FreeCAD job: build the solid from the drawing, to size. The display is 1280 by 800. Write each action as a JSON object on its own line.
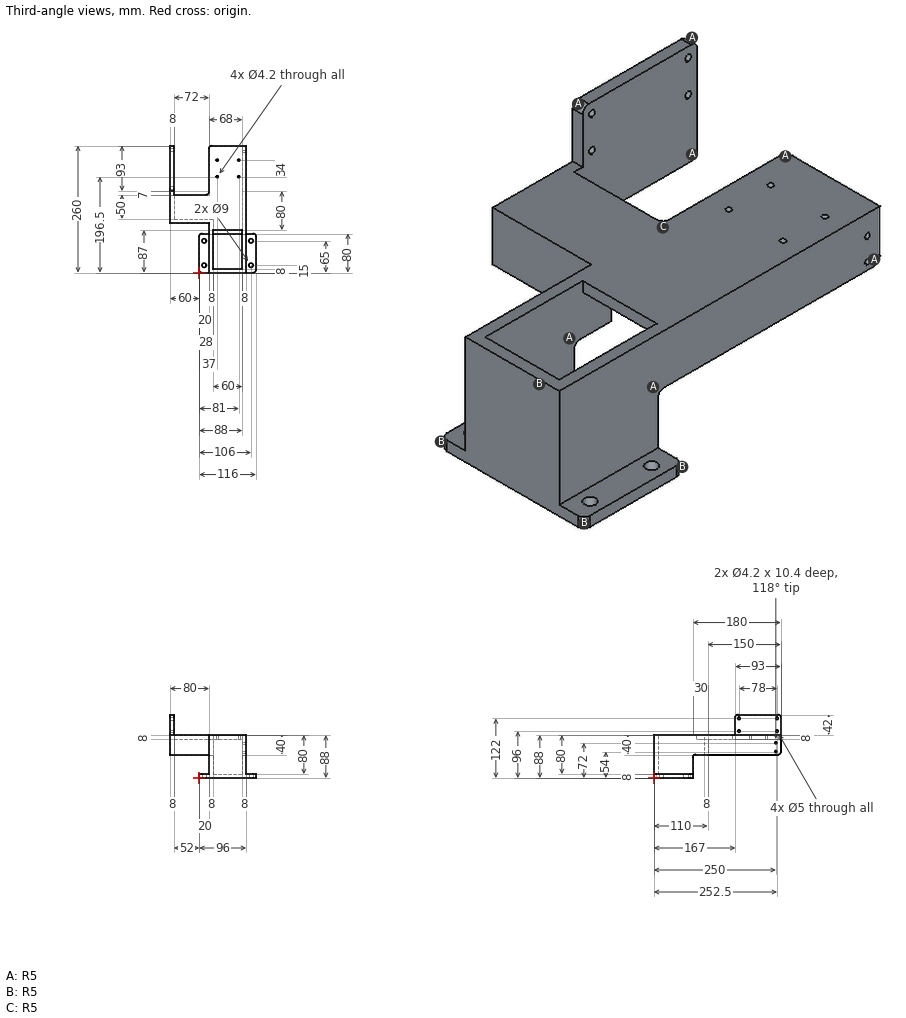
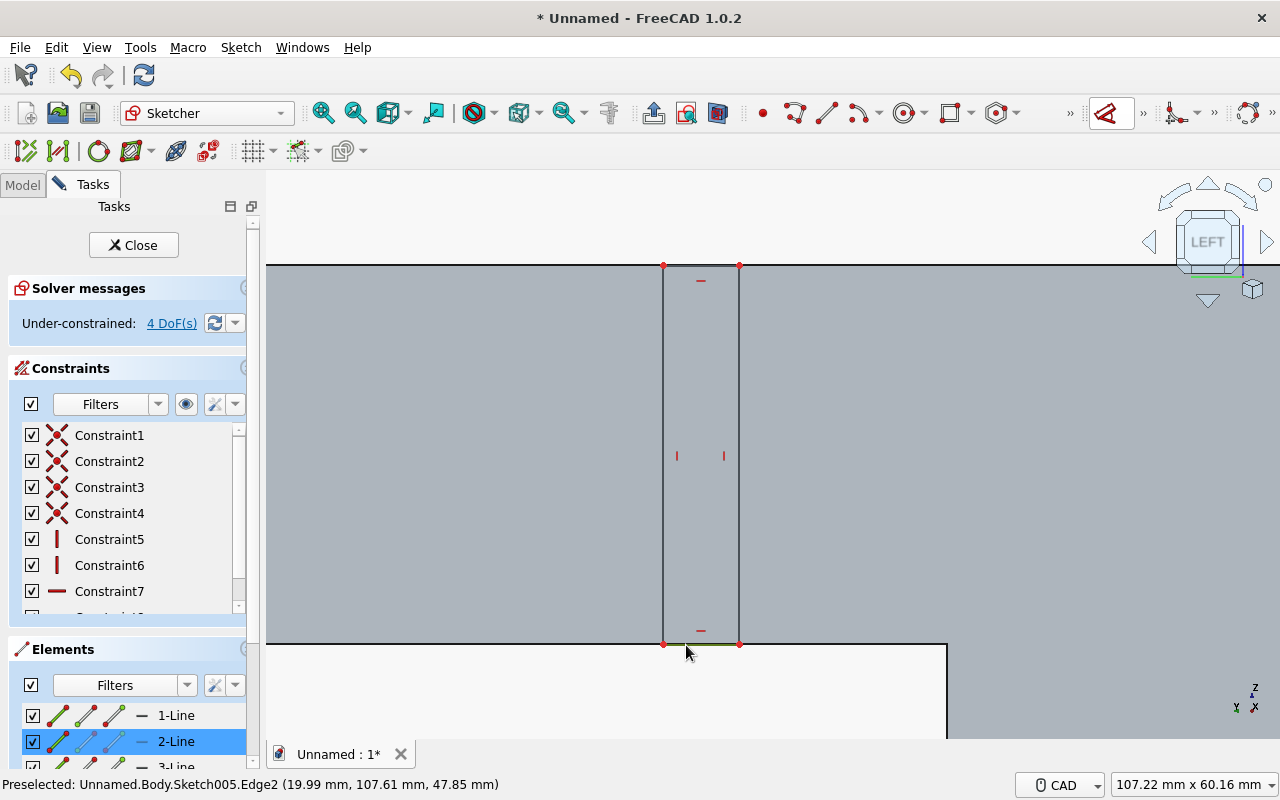
{"action": "left_click", "coordinate": [1128, 114]}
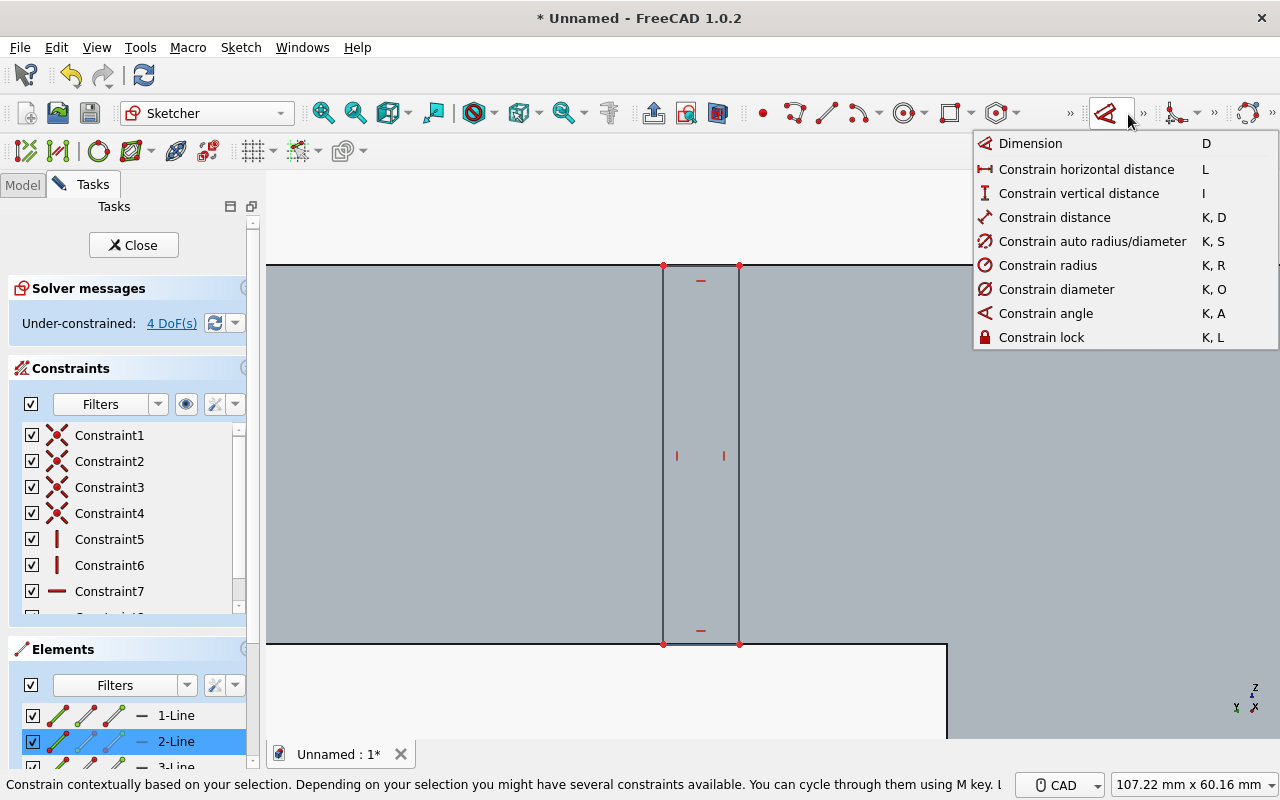
{"action": "left_click", "coordinate": [1126, 169]}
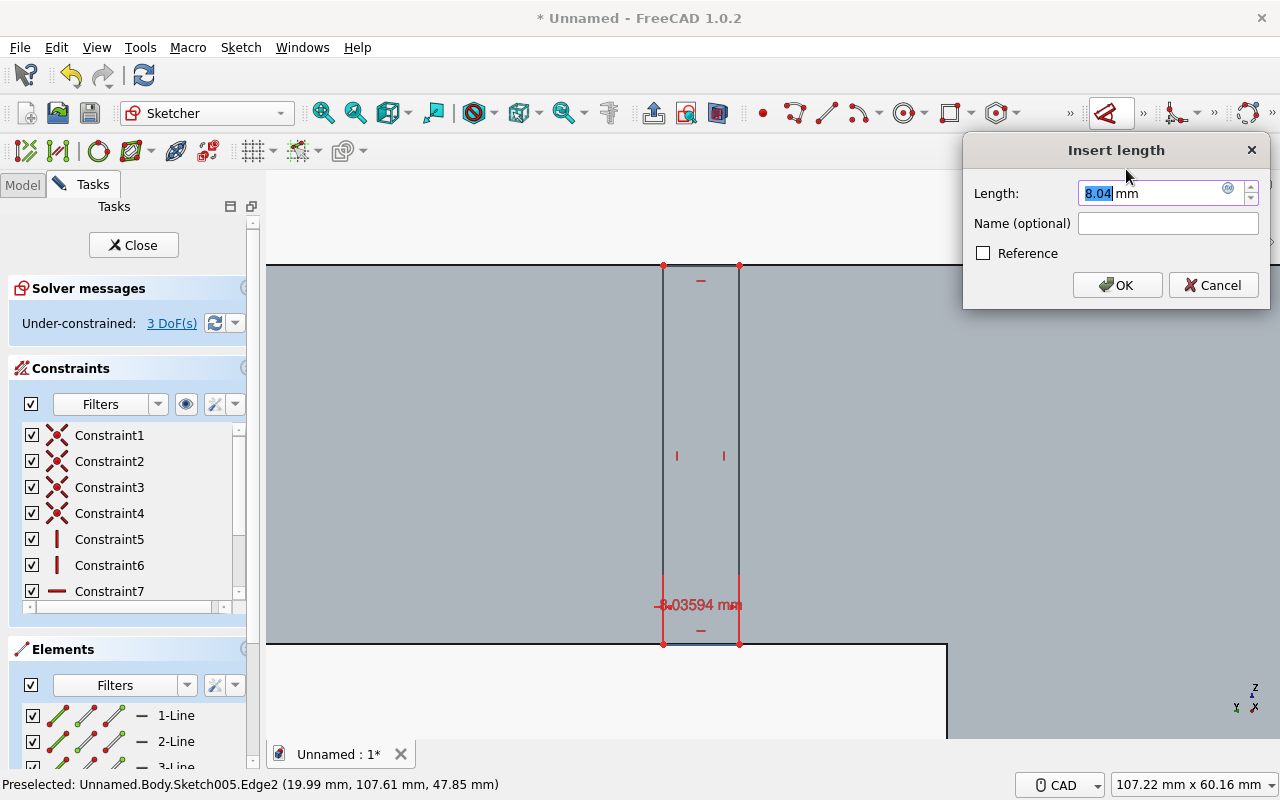
{"action": "type", "text": "8"}
{"action": "key", "text": "Return"}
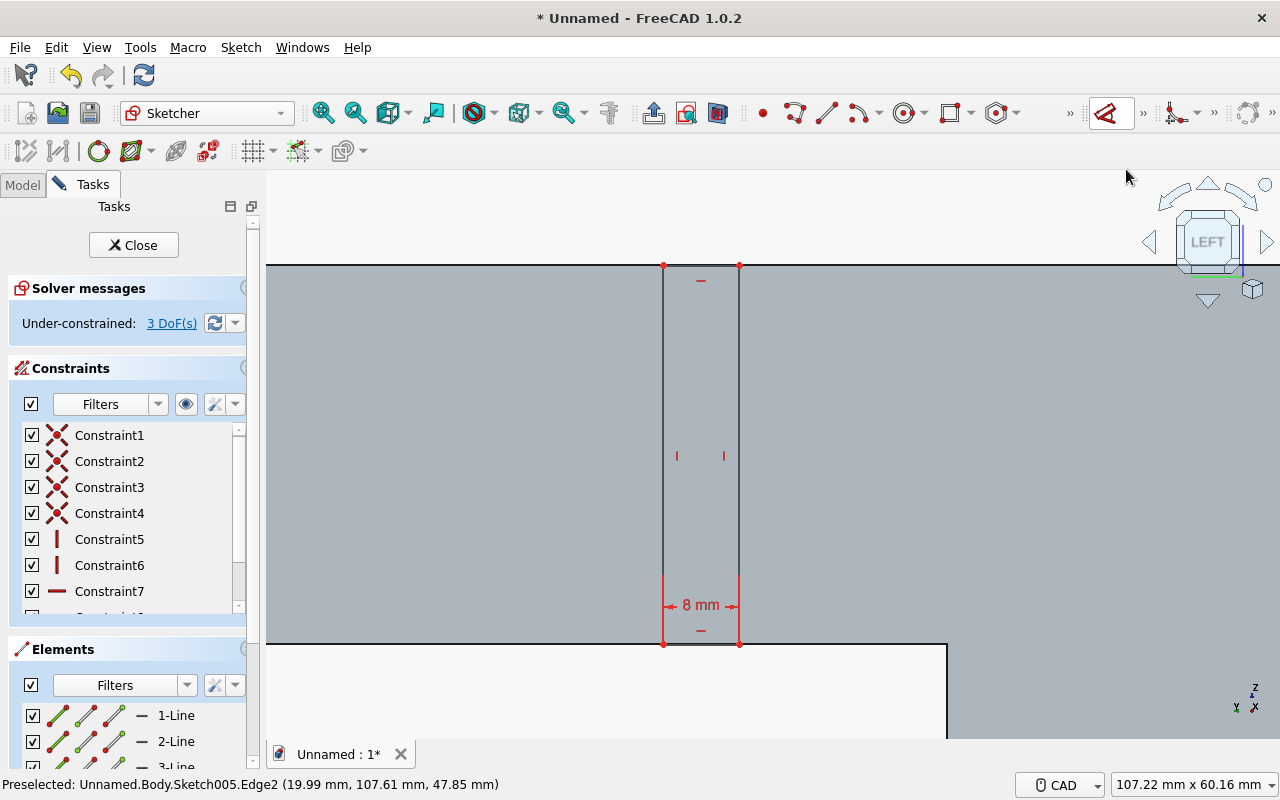
{"action": "left_click", "coordinate": [663, 380]}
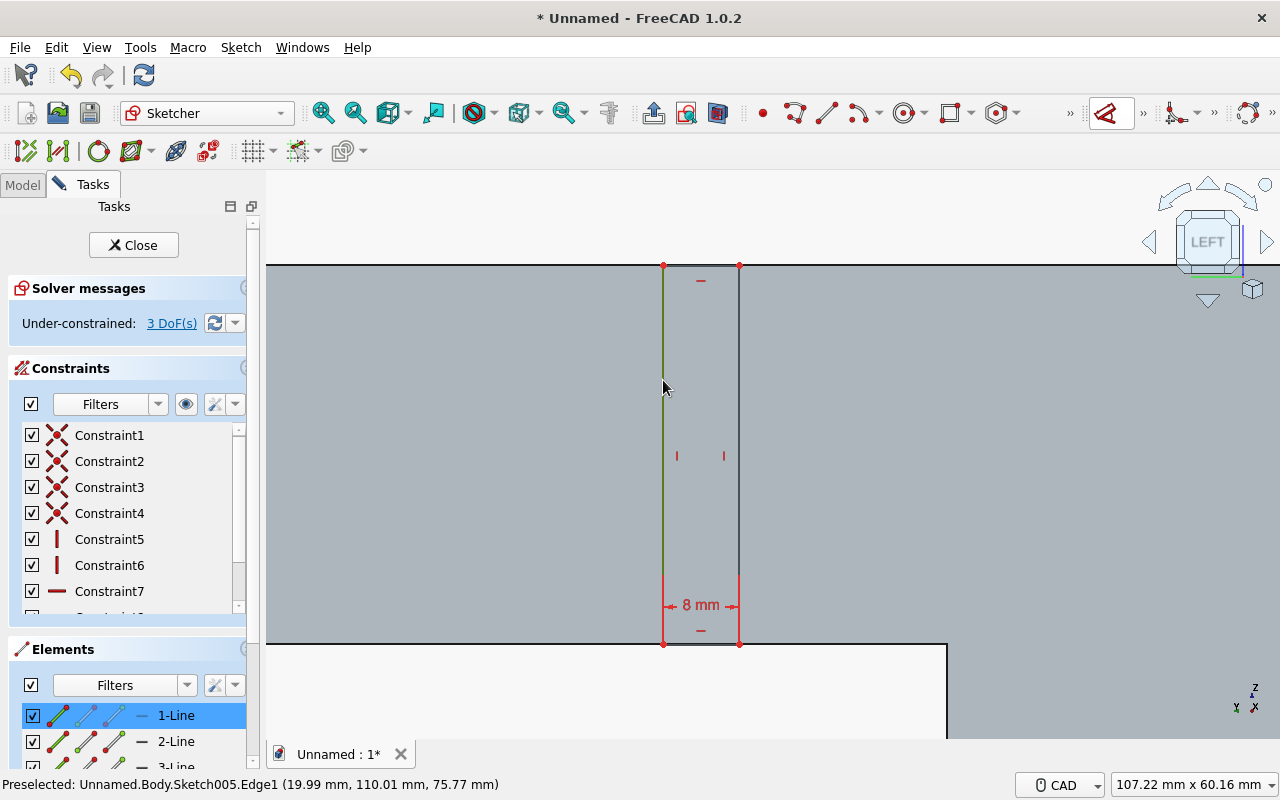
{"action": "left_click", "coordinate": [1128, 114]}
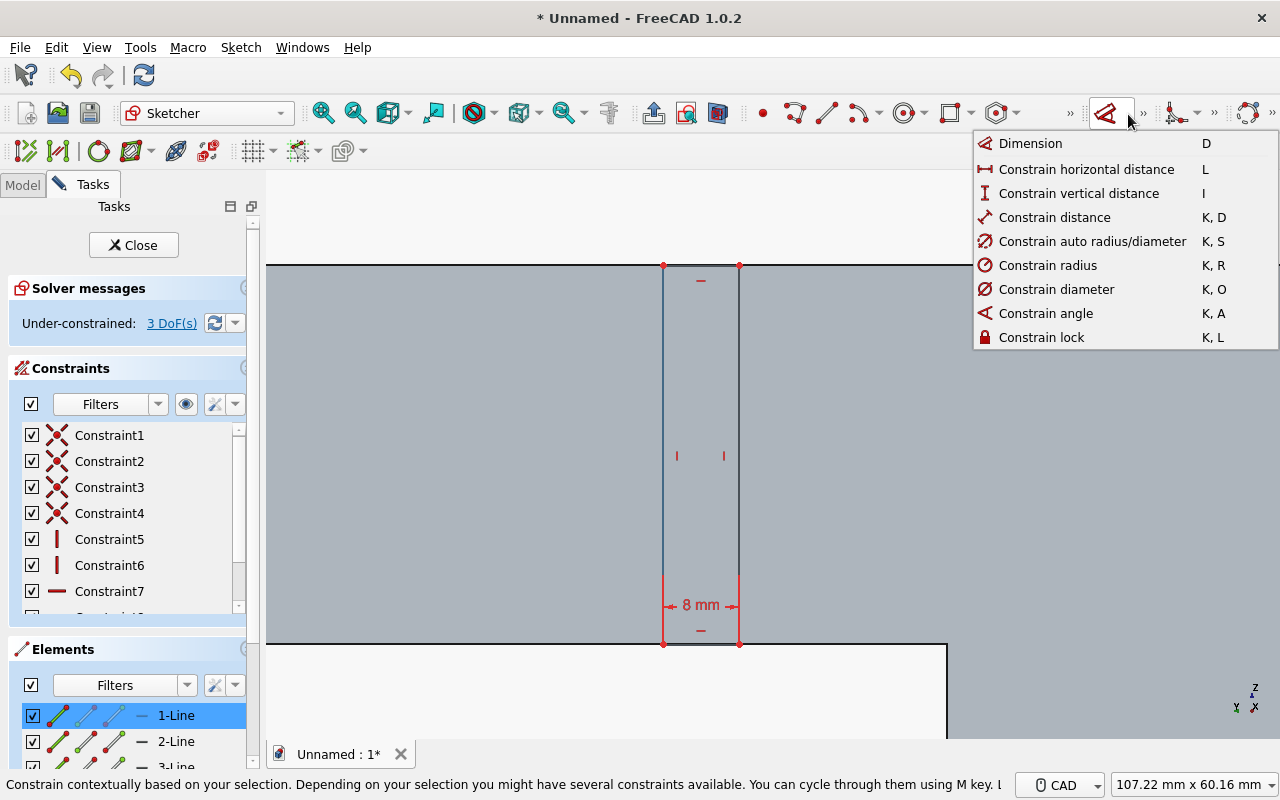
{"action": "left_click", "coordinate": [1126, 193]}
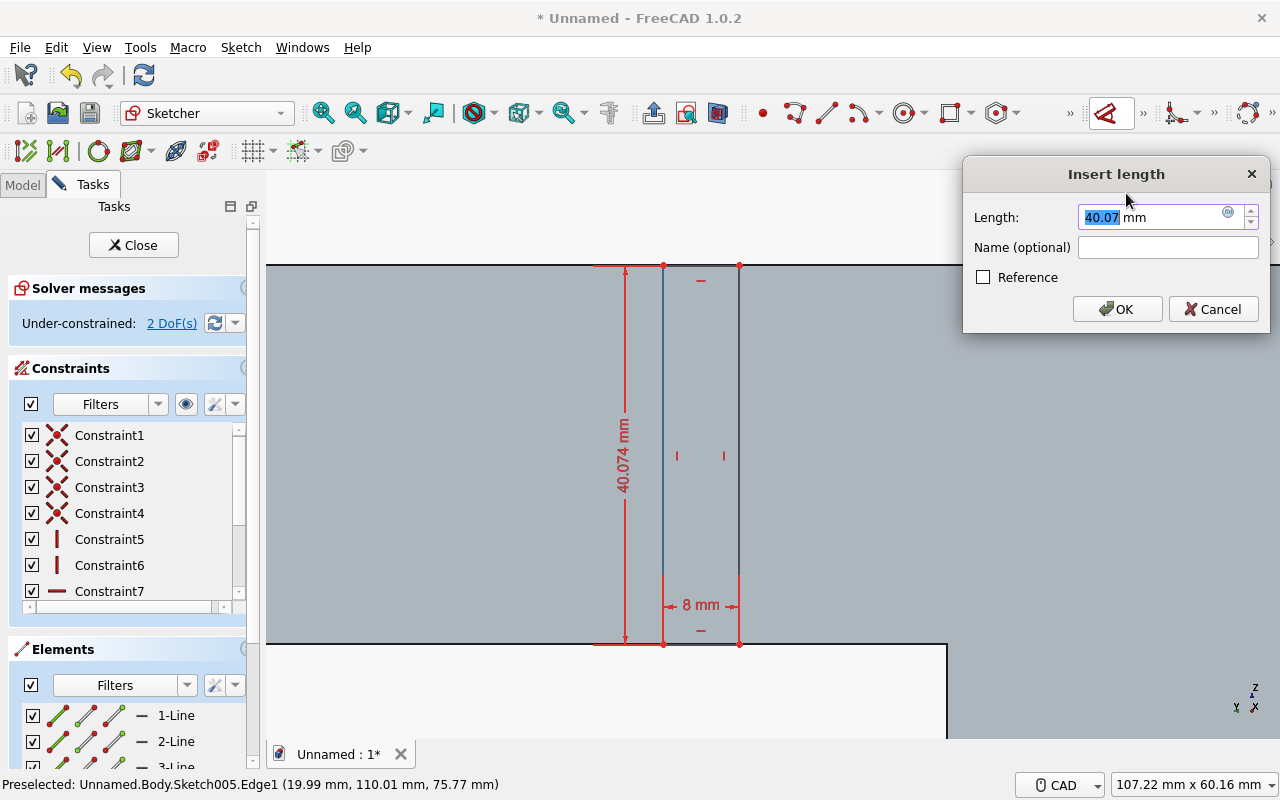
{"action": "type", "text": "40"}
{"action": "key", "text": "Return"}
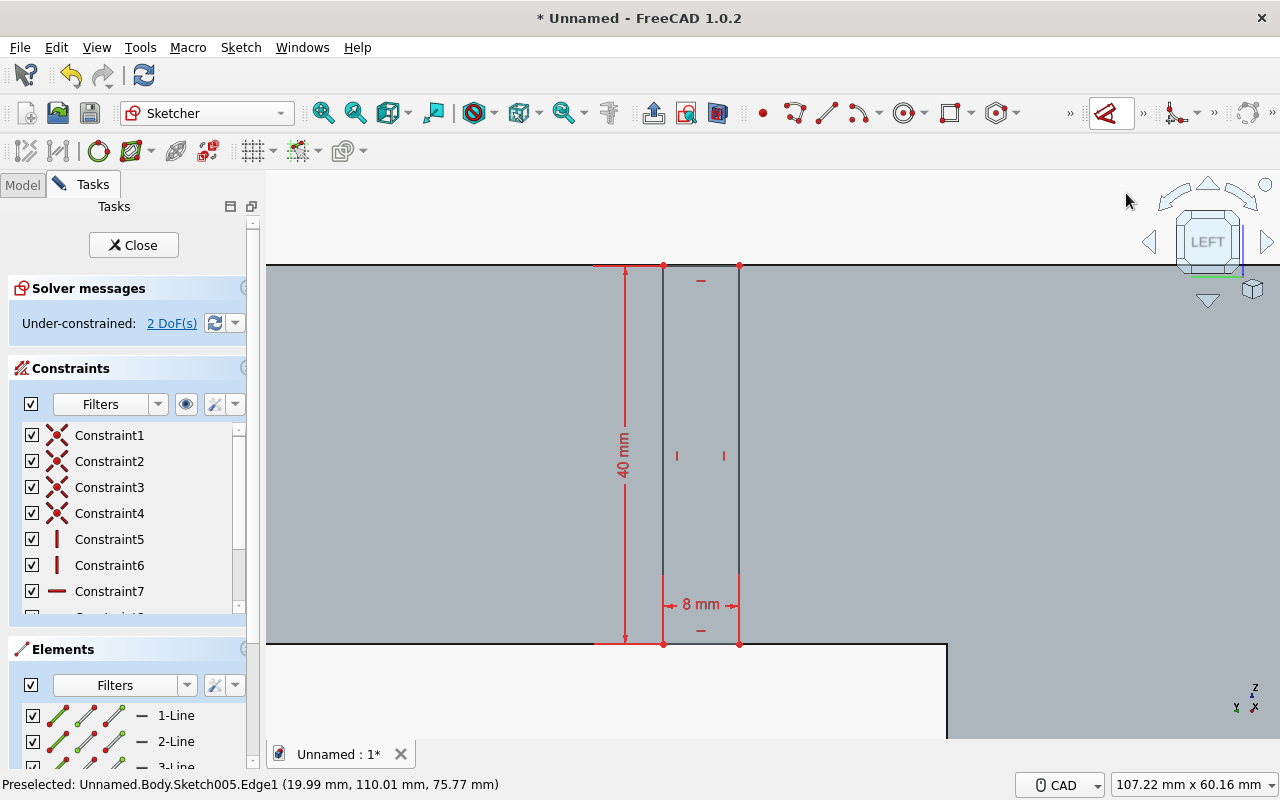
{"action": "left_click", "coordinate": [663, 266]}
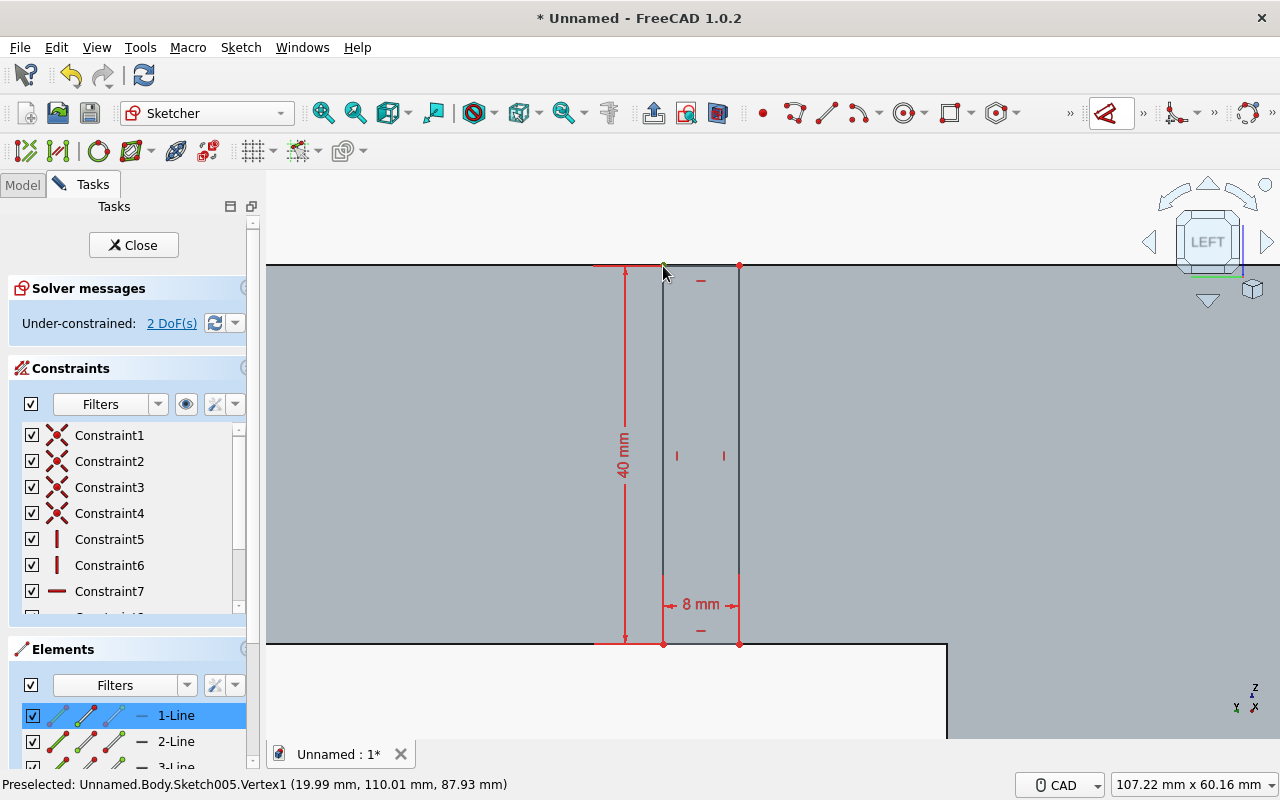
{"action": "left_click", "coordinate": [1128, 114]}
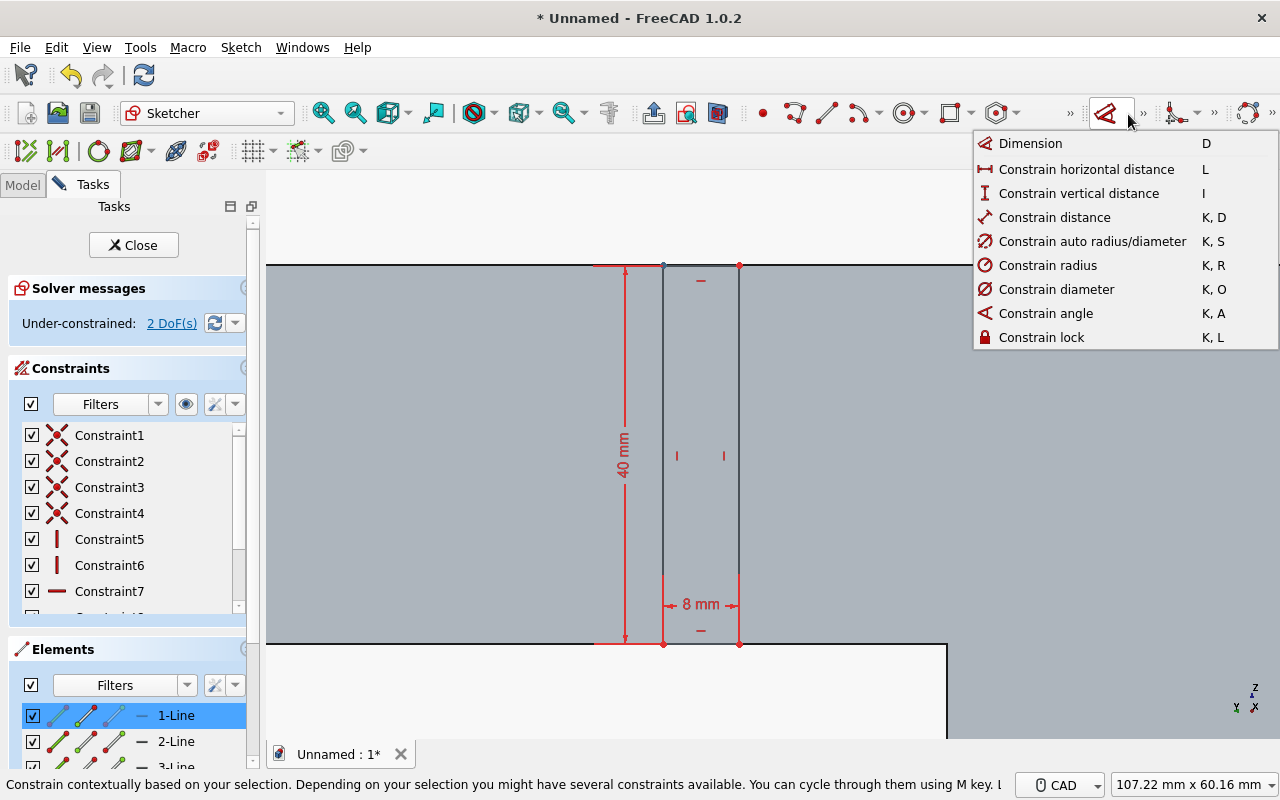
{"action": "left_click", "coordinate": [1126, 193]}